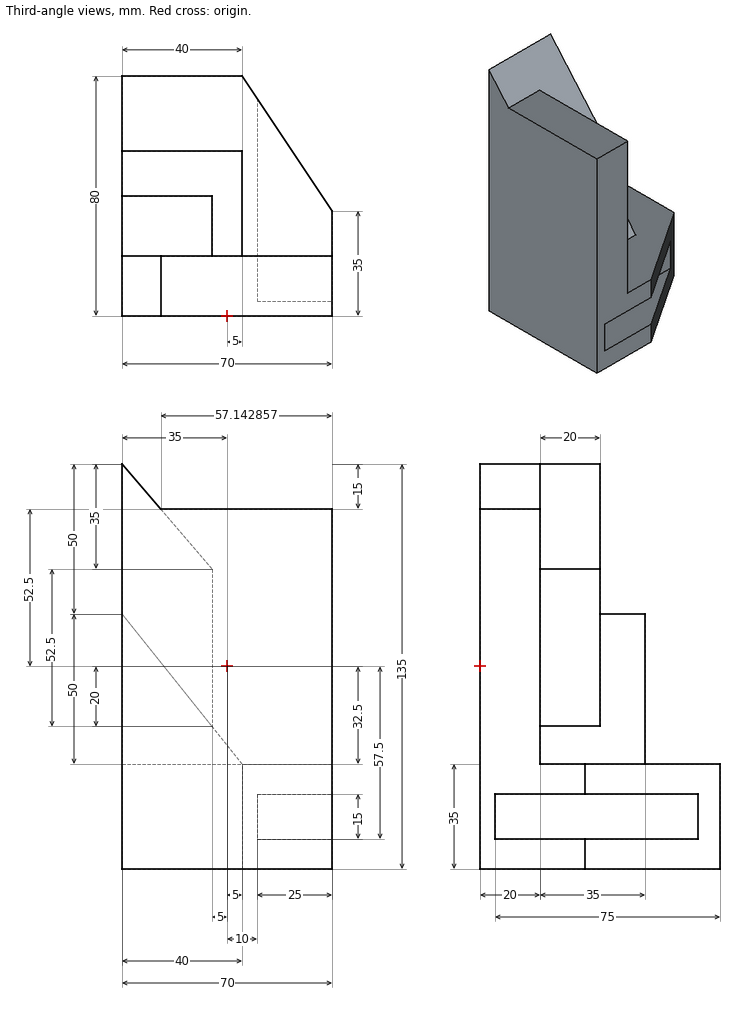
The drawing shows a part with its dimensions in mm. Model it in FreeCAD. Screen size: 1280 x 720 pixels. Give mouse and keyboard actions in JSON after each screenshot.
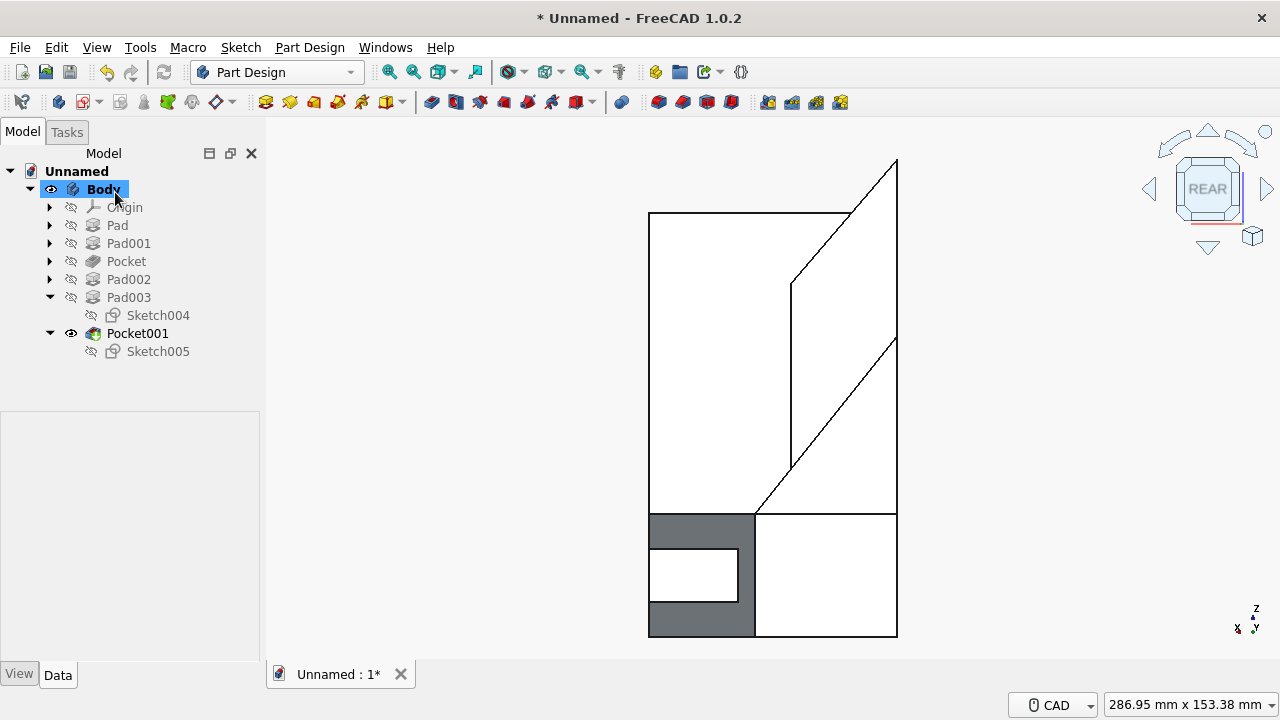
{"action": "key", "text": "0"}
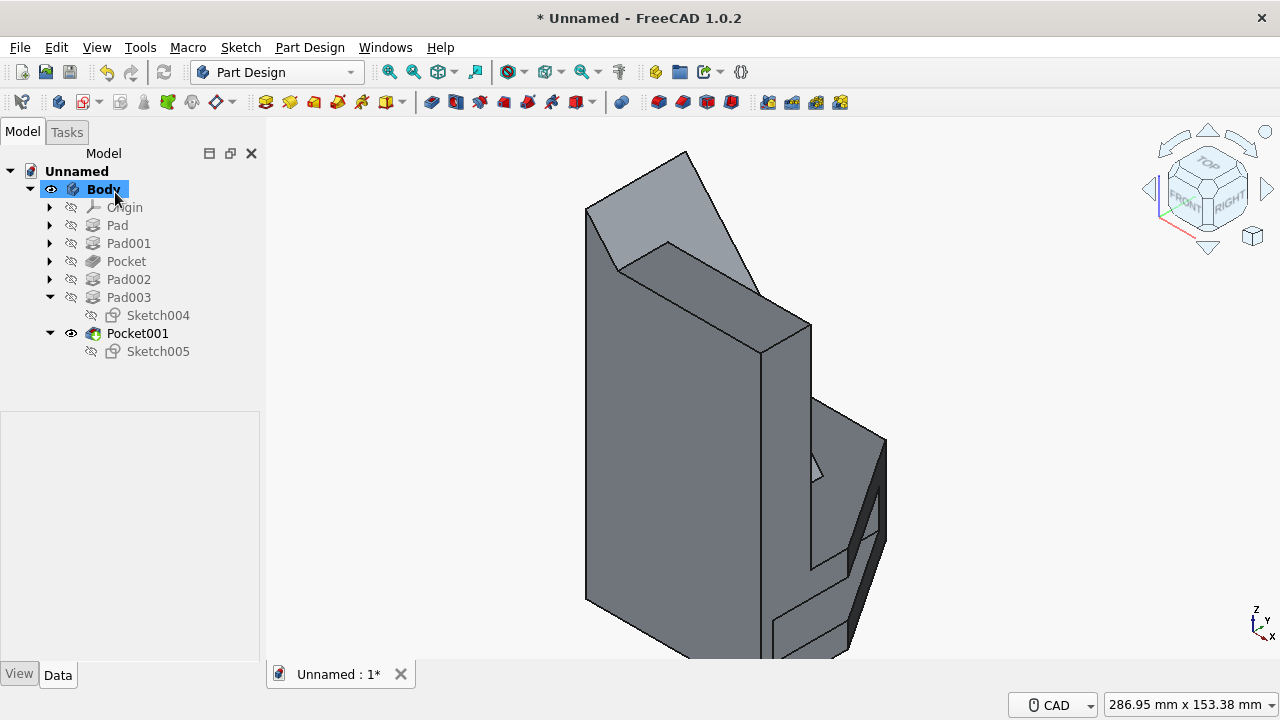
{"action": "left_click", "coordinate": [390, 72]}